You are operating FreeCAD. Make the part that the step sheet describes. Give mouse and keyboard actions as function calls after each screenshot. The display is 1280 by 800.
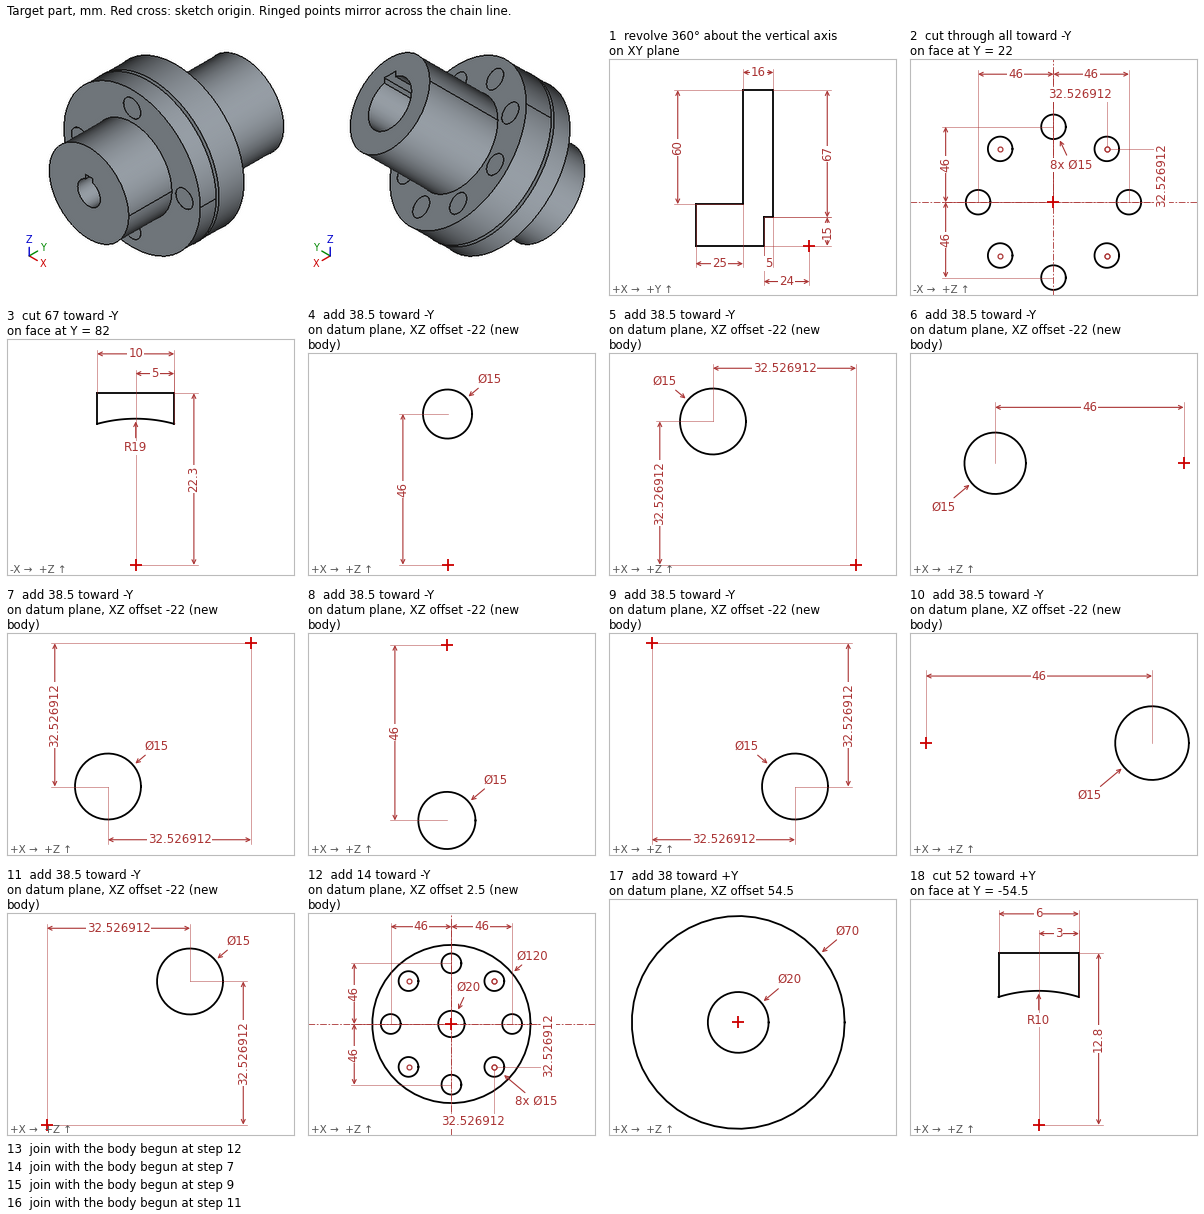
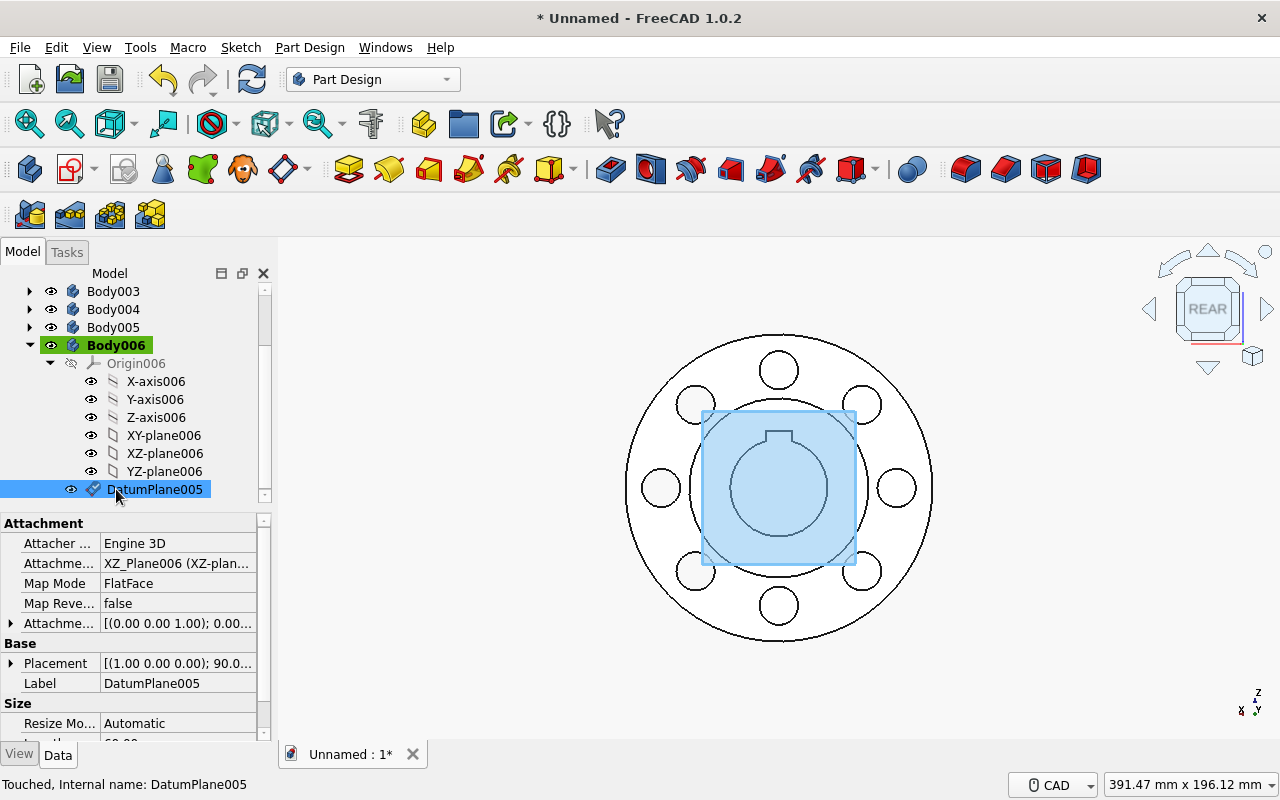
click(70, 170)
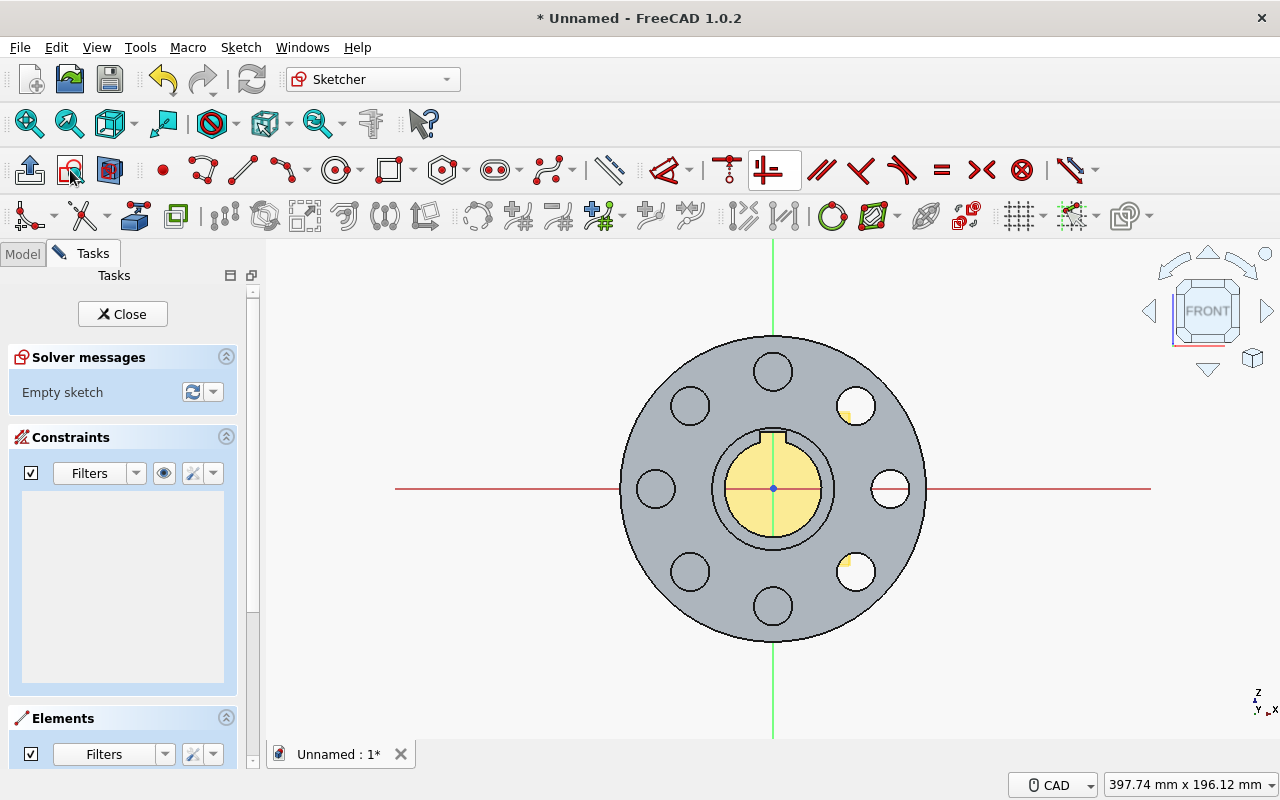
scroll(875, 582, up, 11)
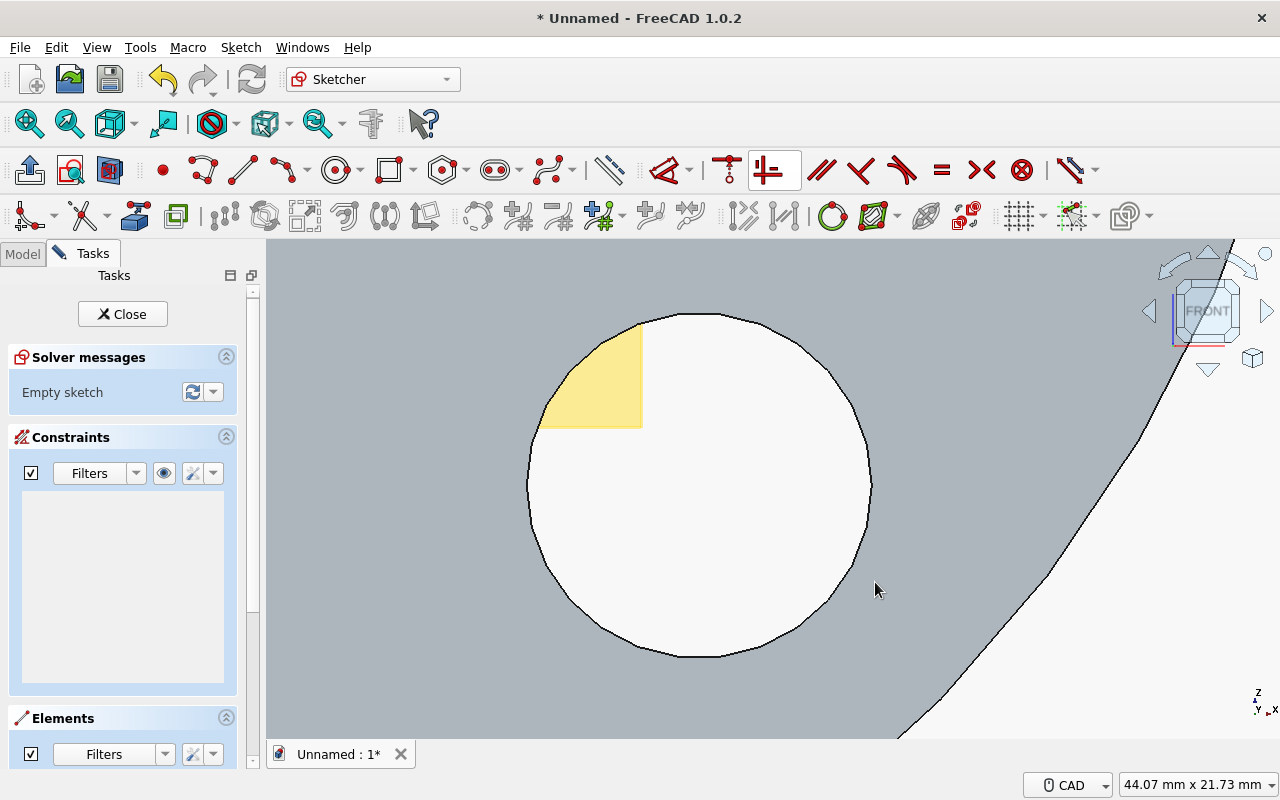
click(336, 170)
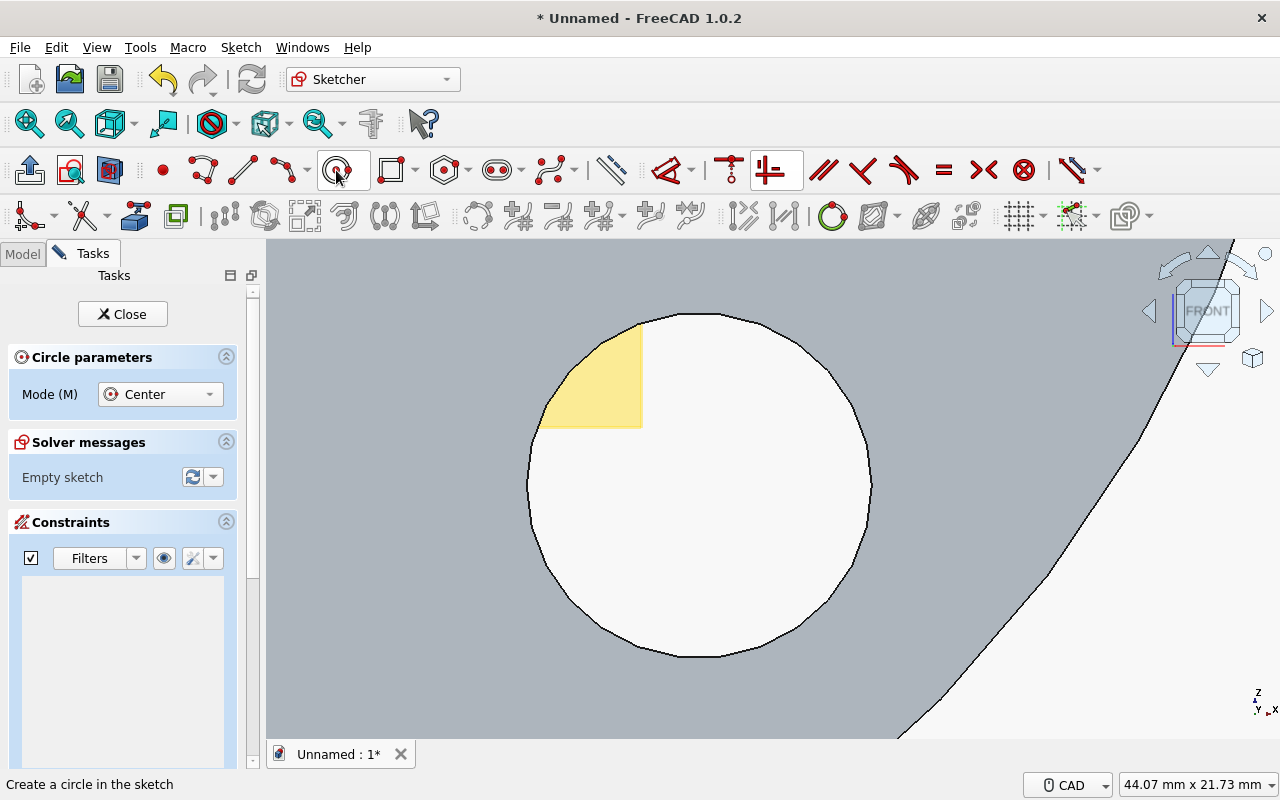
click(699, 486)
click(821, 364)
key(Escape)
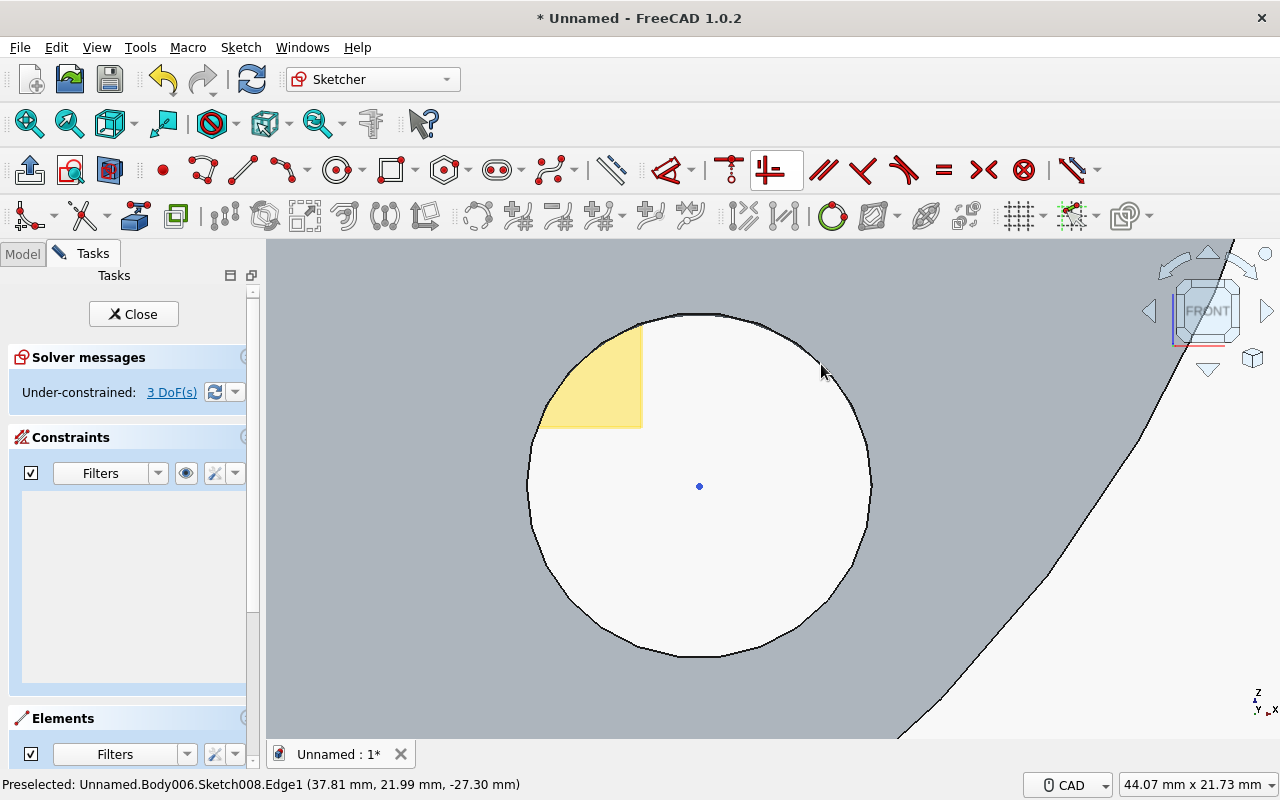
click(666, 170)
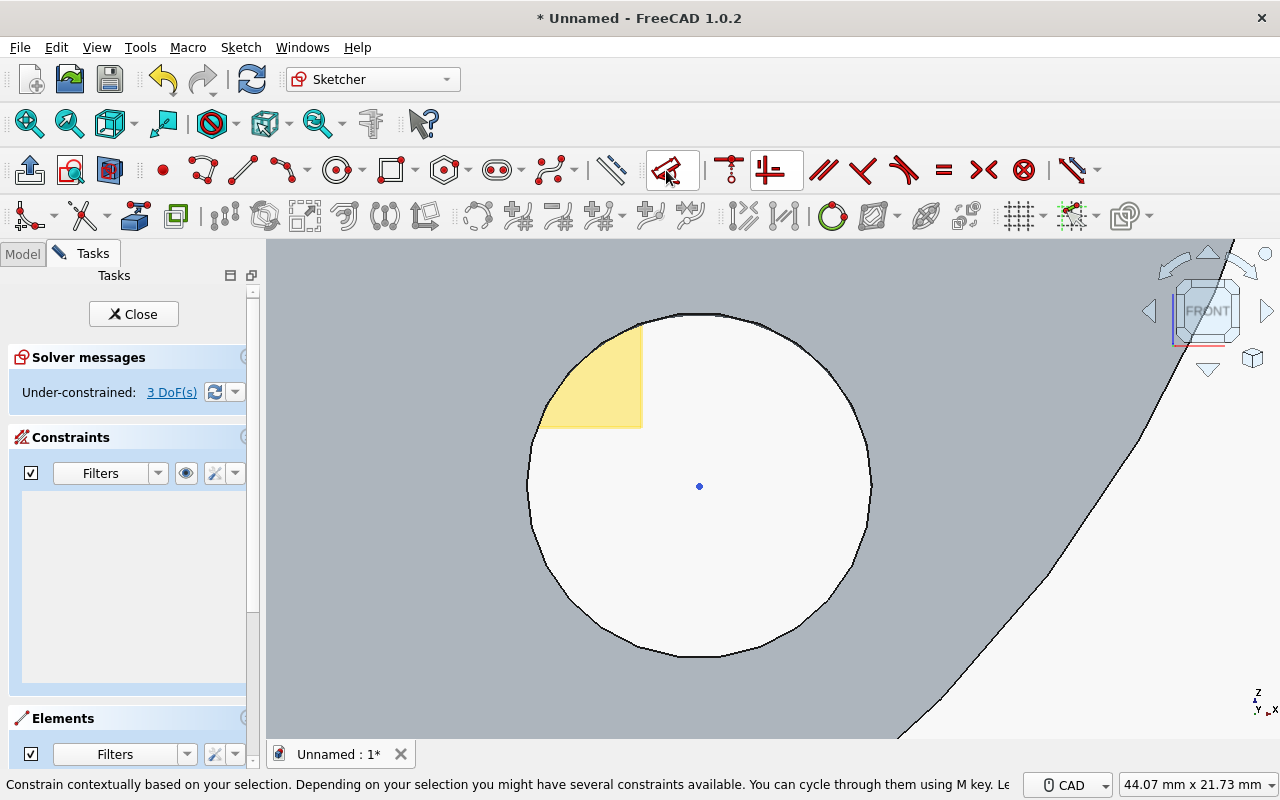
click(821, 365)
click(844, 342)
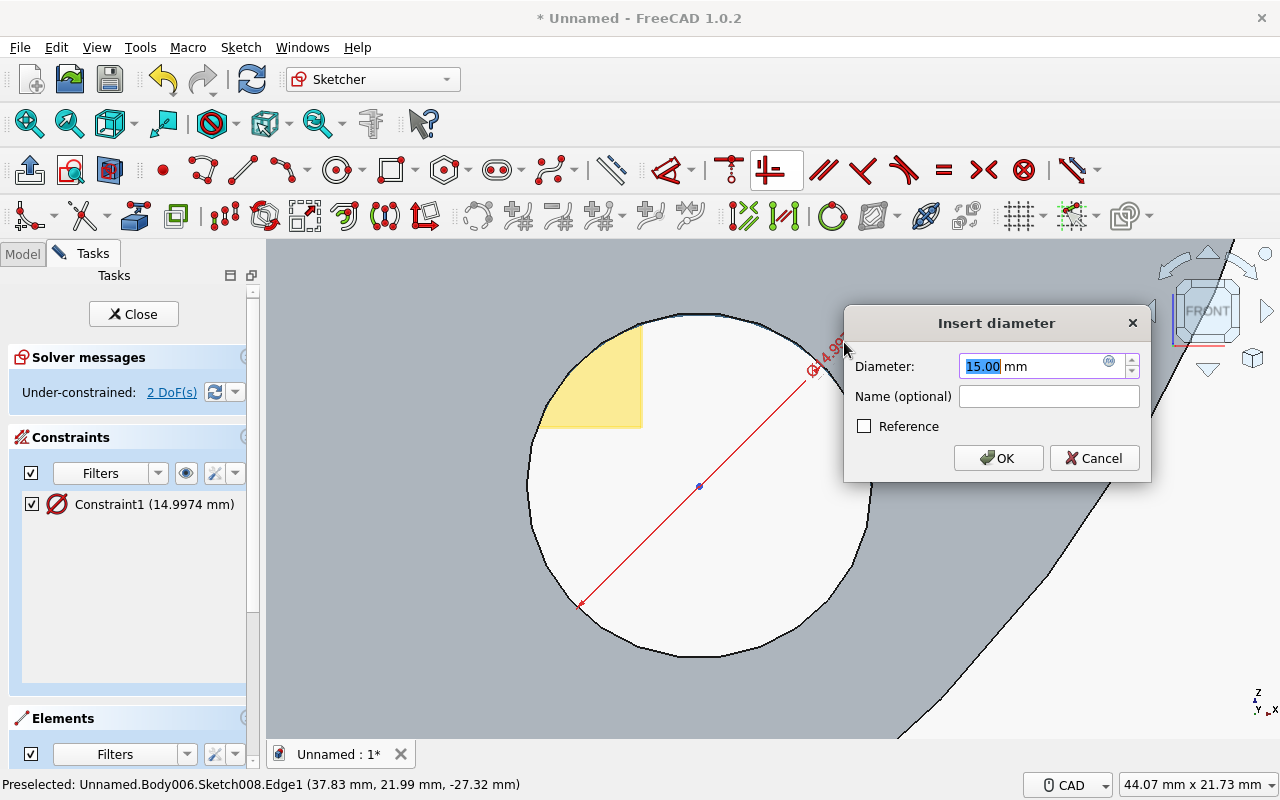
text(15)
key(Return)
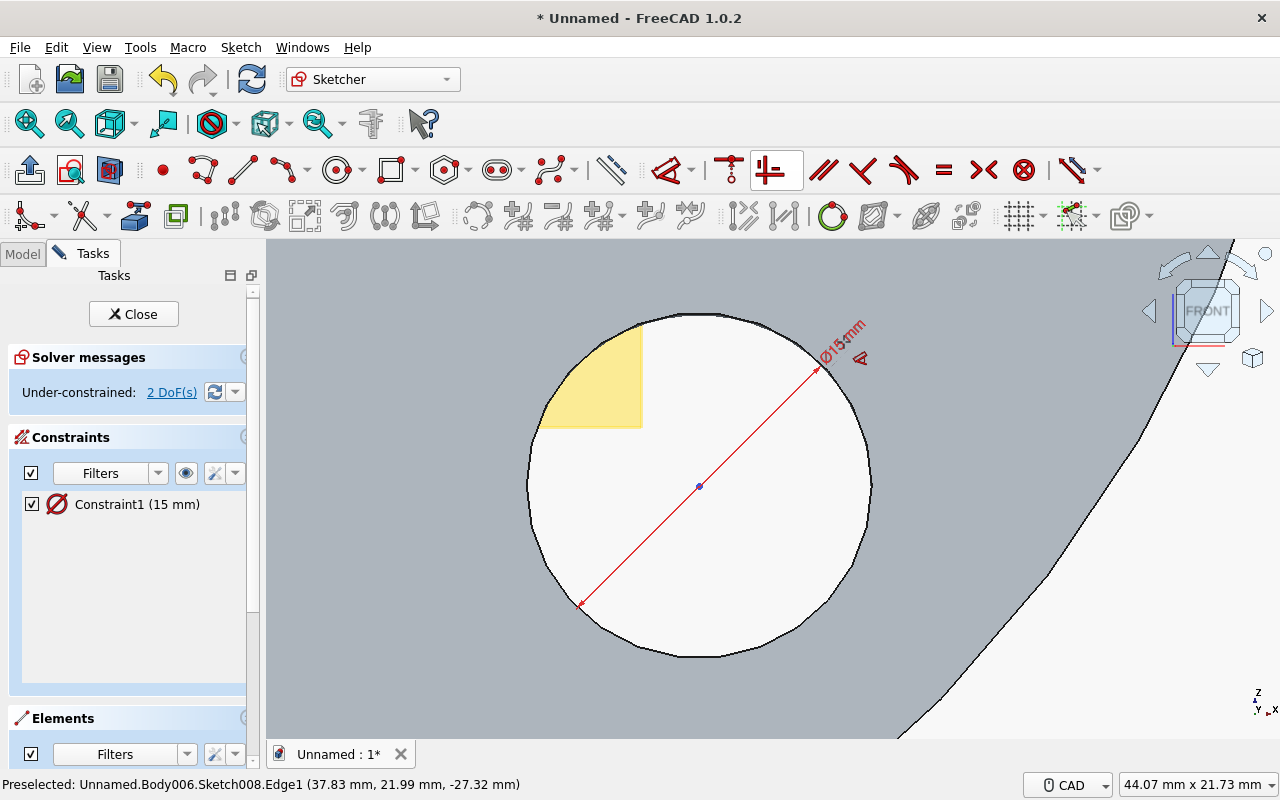
click(699, 487)
click(496, 521)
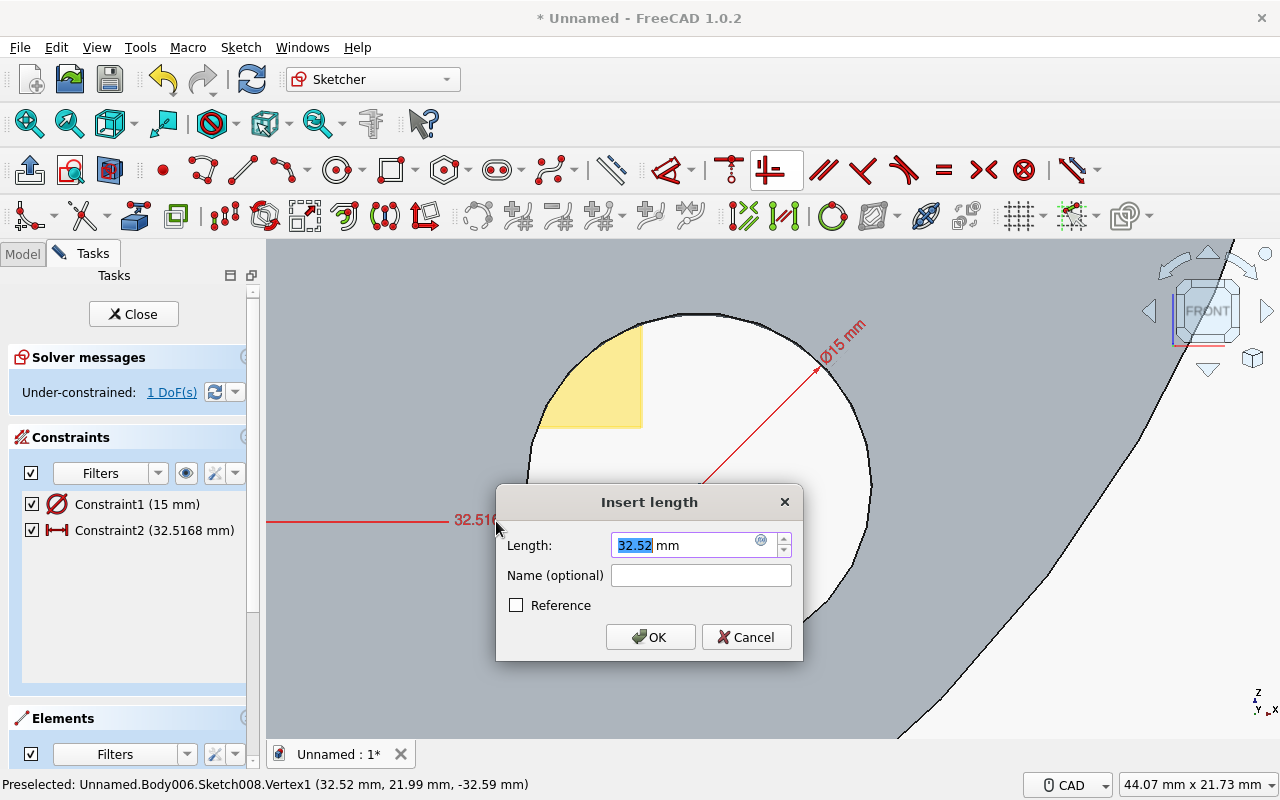
text(32.526912)
key(Return)